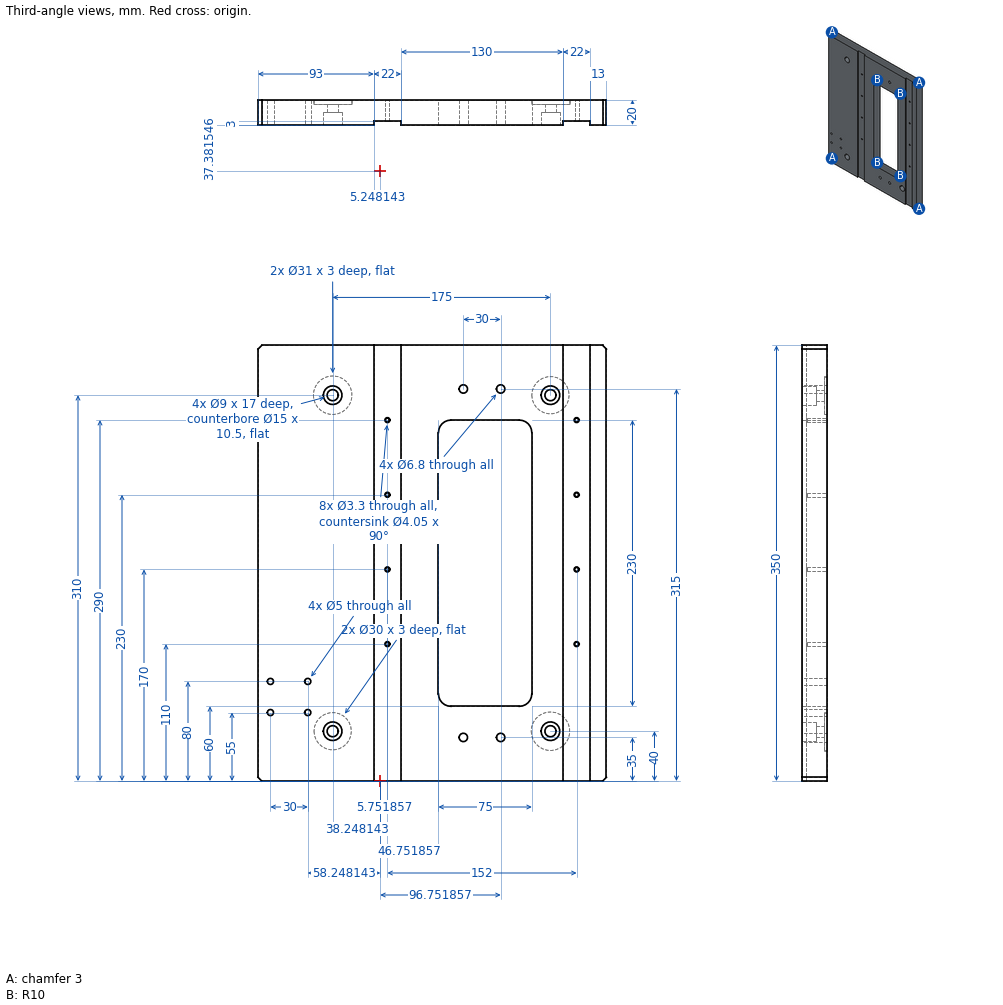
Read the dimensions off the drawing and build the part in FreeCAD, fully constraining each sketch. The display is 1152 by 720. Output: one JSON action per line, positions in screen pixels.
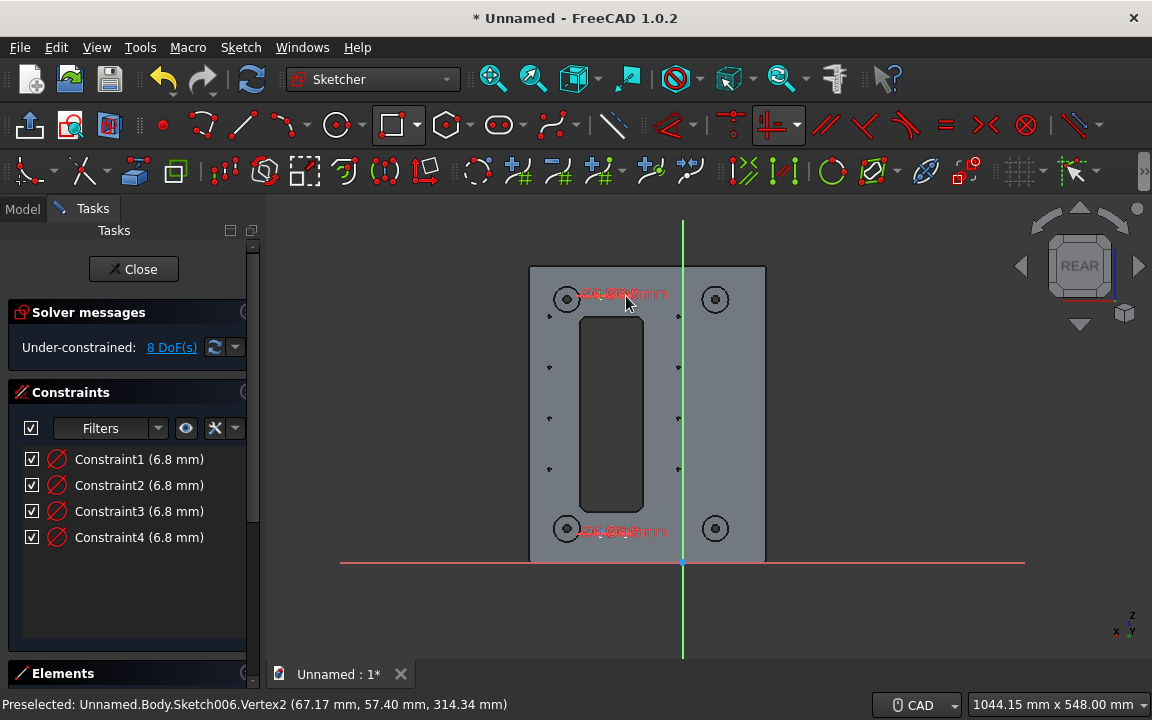
{"action": "left_click", "coordinate": [800, 126]}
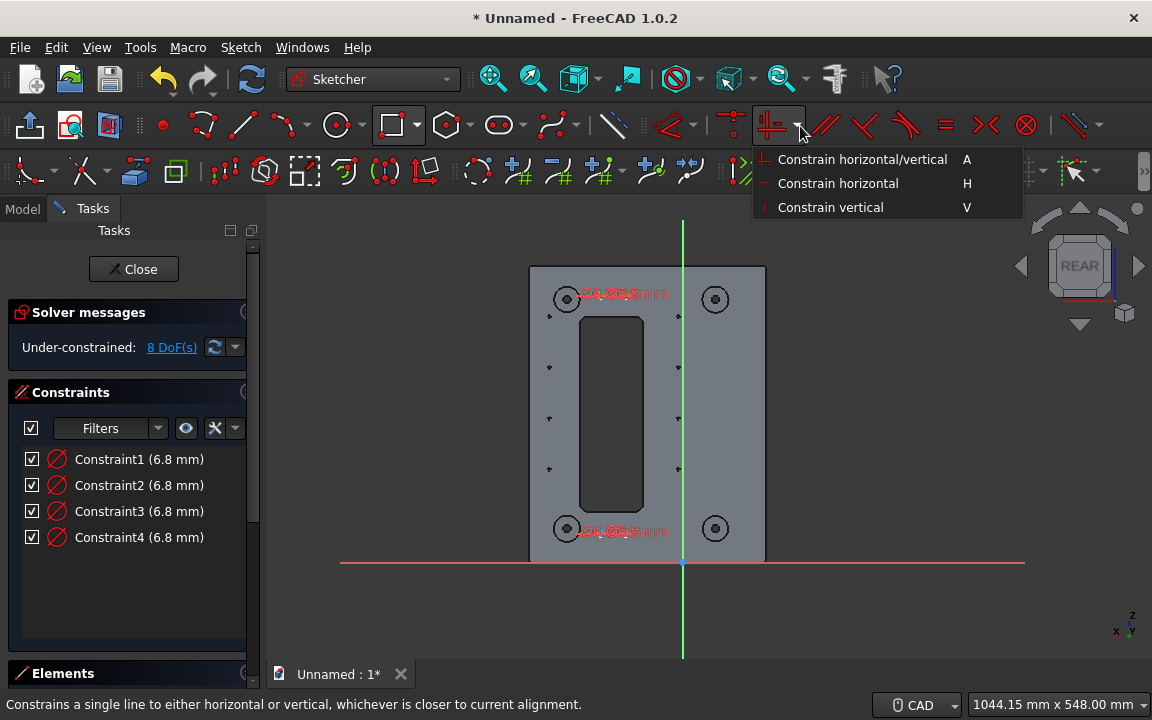
{"action": "left_click", "coordinate": [888, 183]}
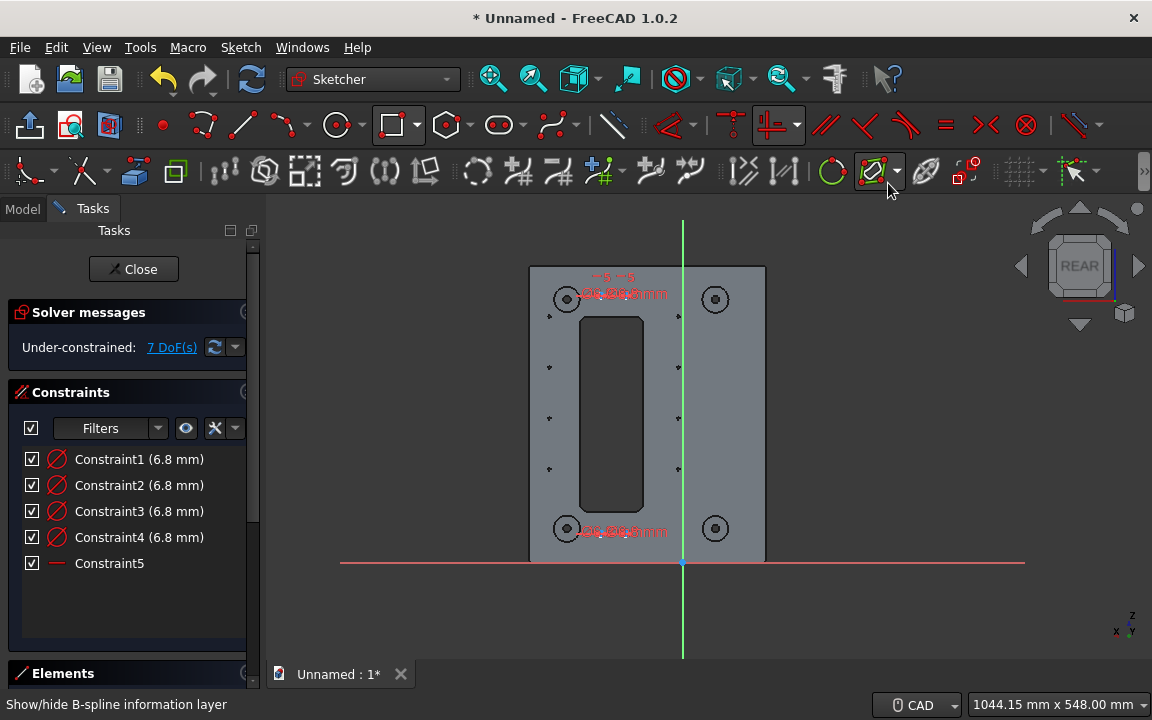
{"action": "left_click", "coordinate": [601, 296]}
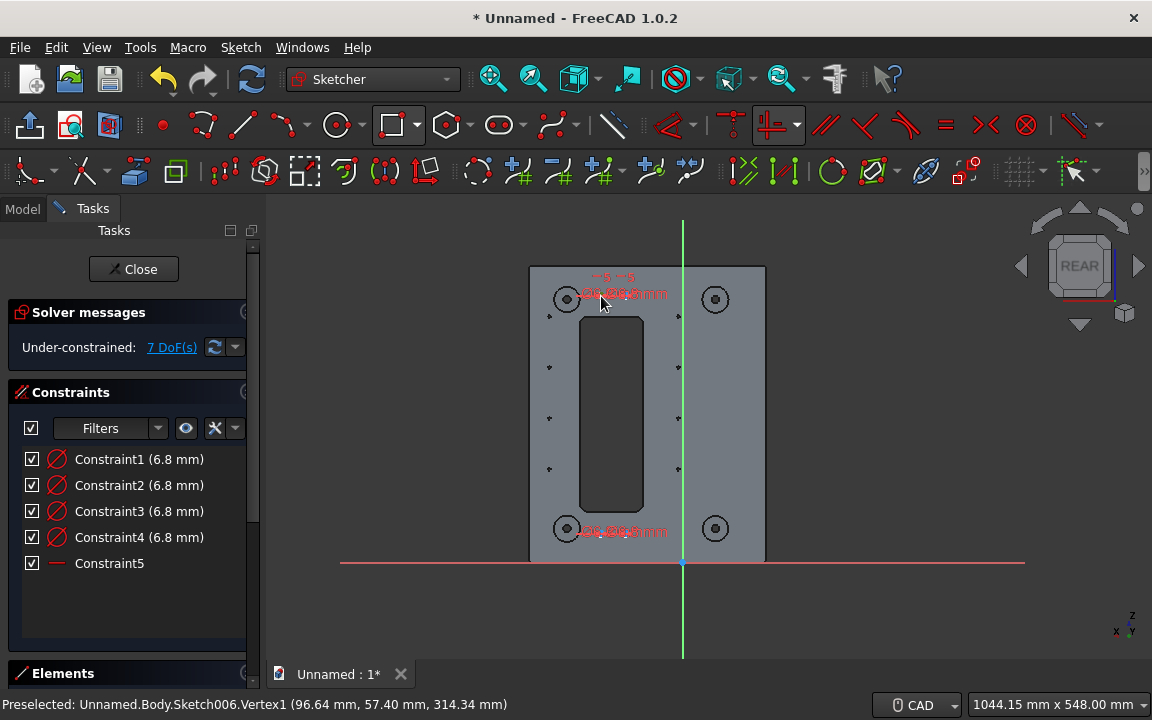
{"action": "left_click", "coordinate": [601, 534]}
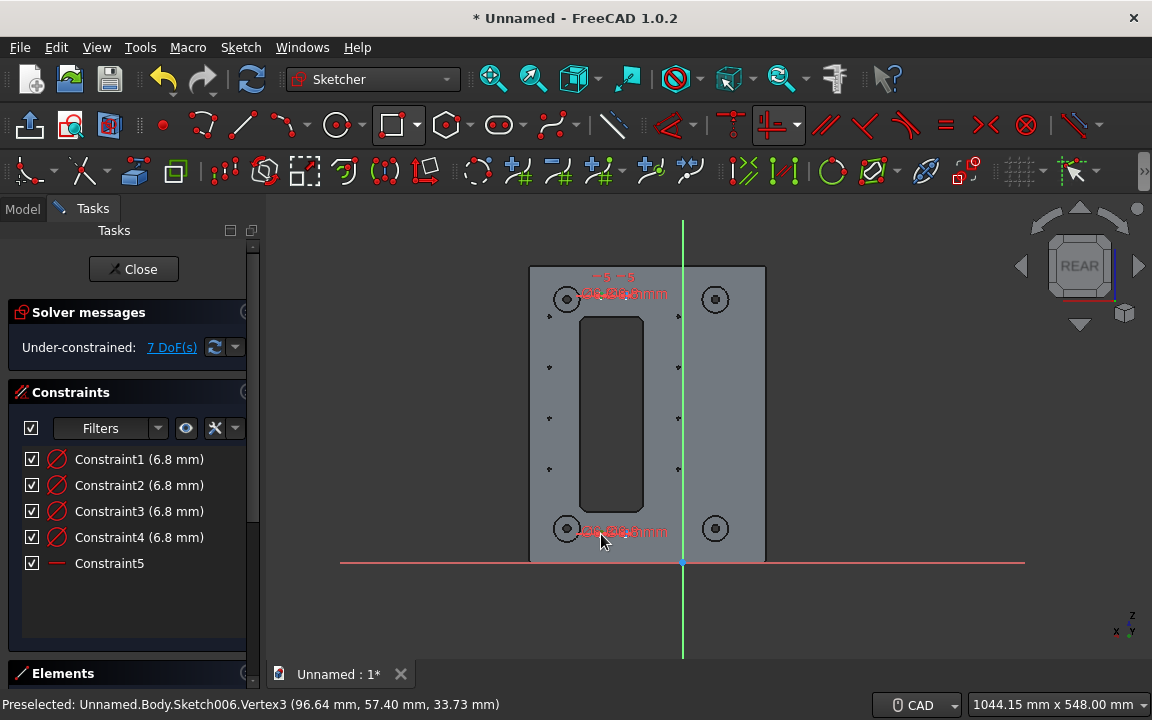
{"action": "key", "text": "v"}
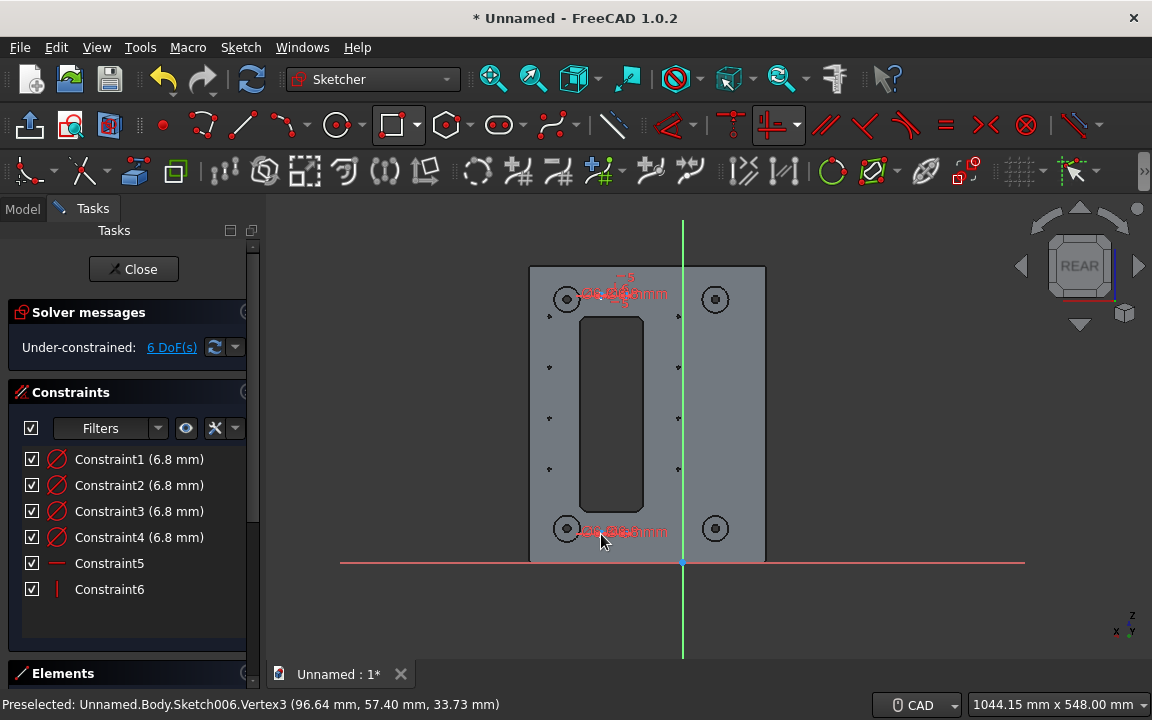
{"action": "left_click", "coordinate": [626, 296]}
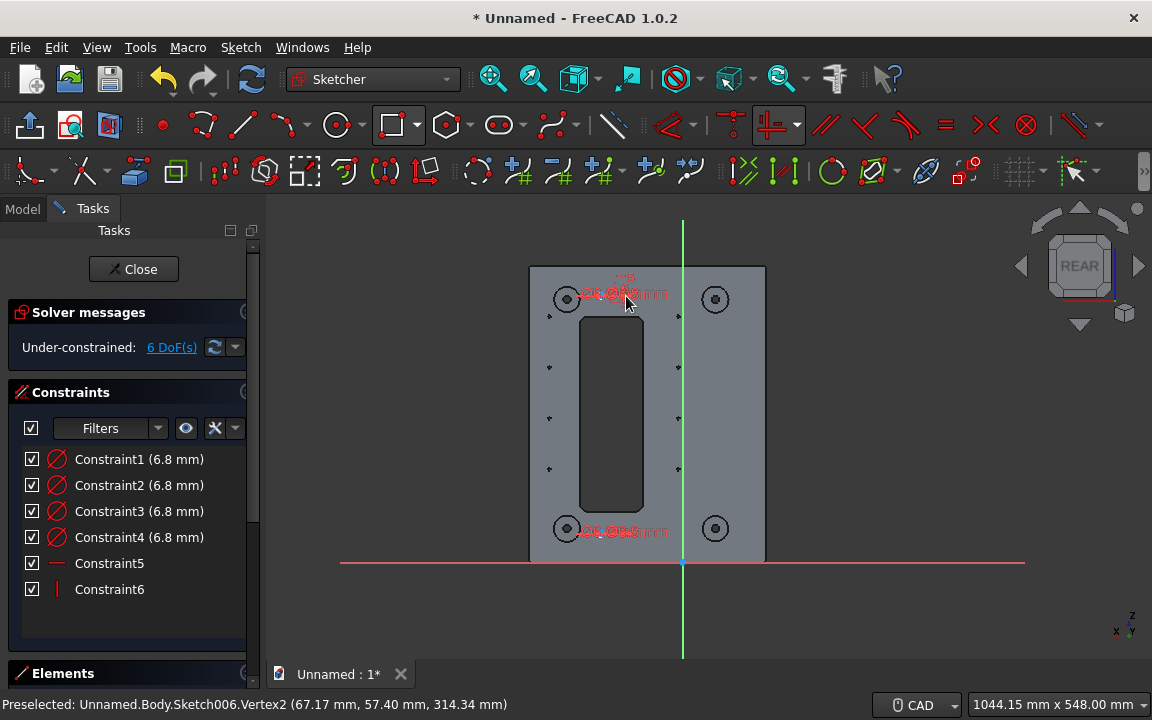
{"action": "scroll", "coordinate": [626, 534], "scroll_direction": "up", "scroll_amount": 4}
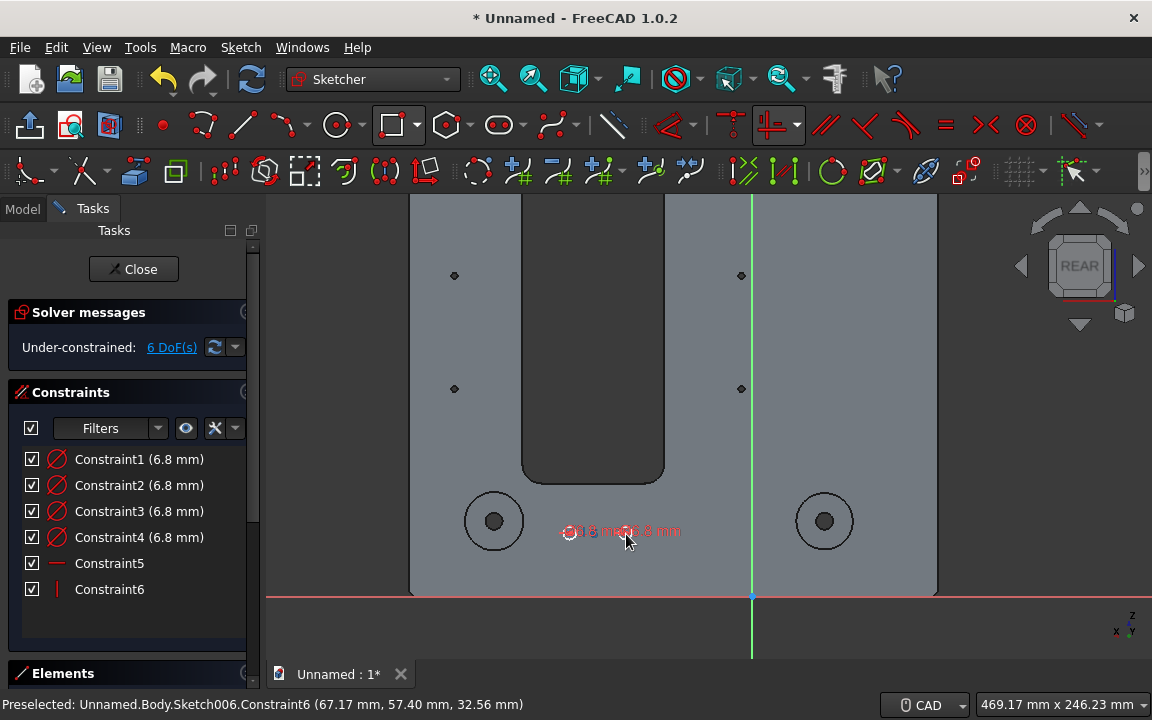
{"action": "left_click", "coordinate": [626, 533]}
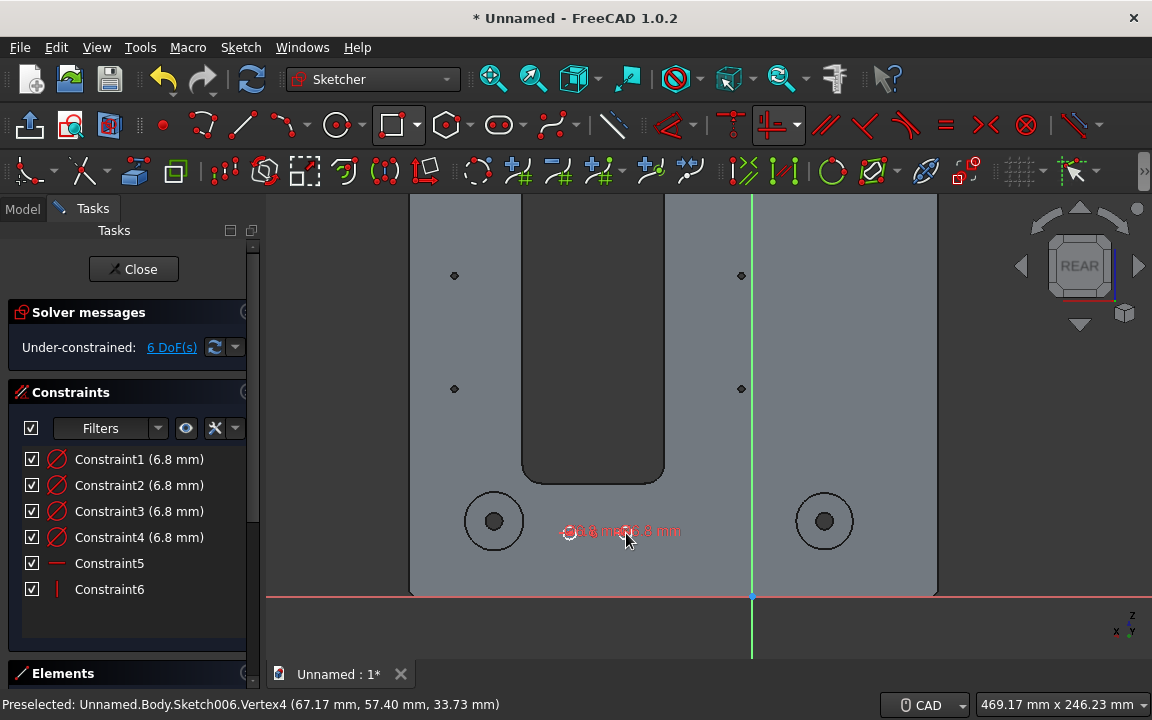
{"action": "left_click", "coordinate": [800, 126]}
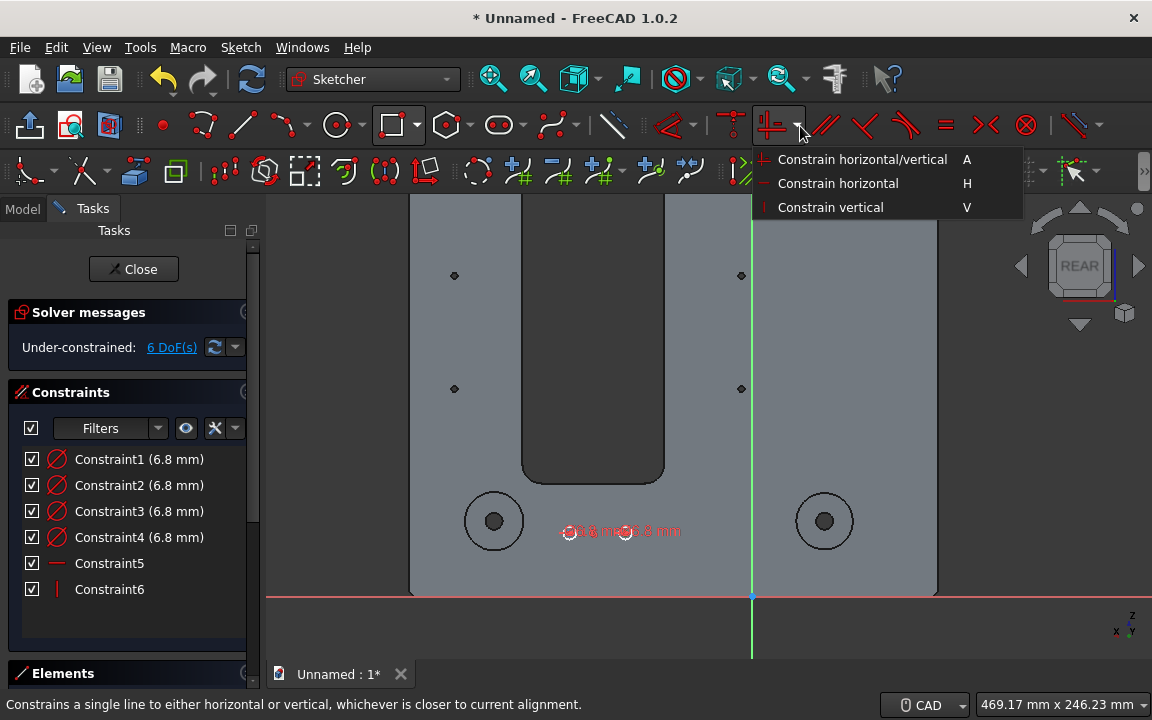
{"action": "left_click", "coordinate": [888, 207]}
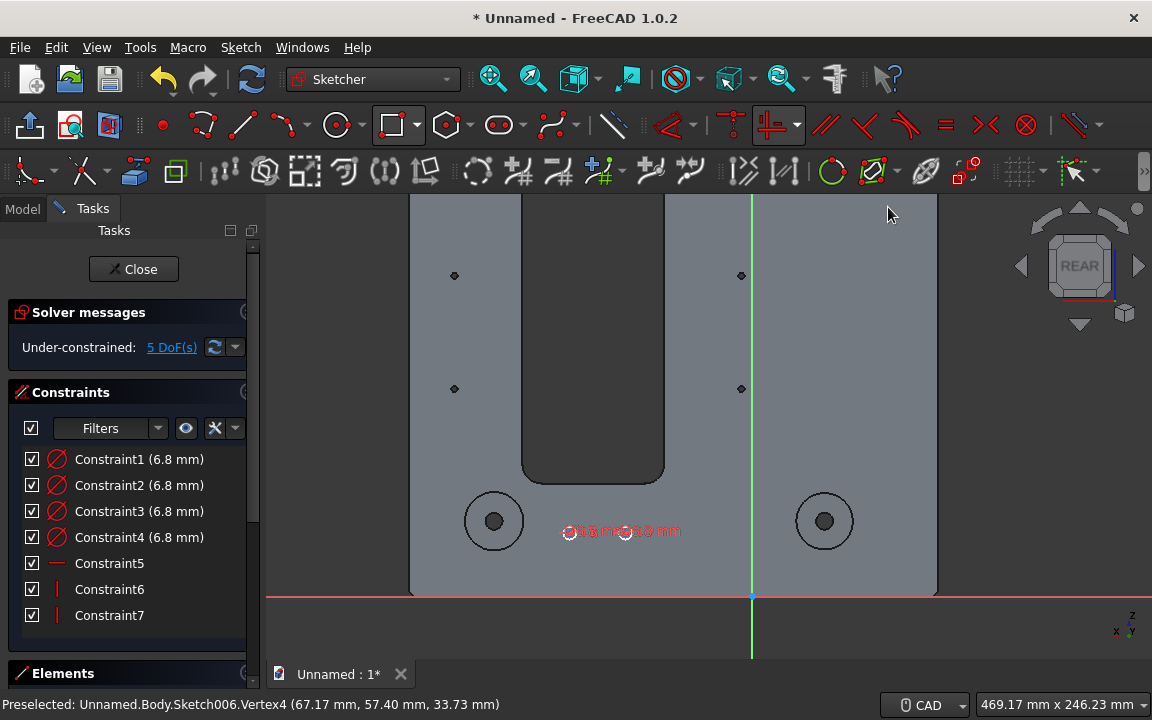
{"action": "left_click", "coordinate": [570, 533]}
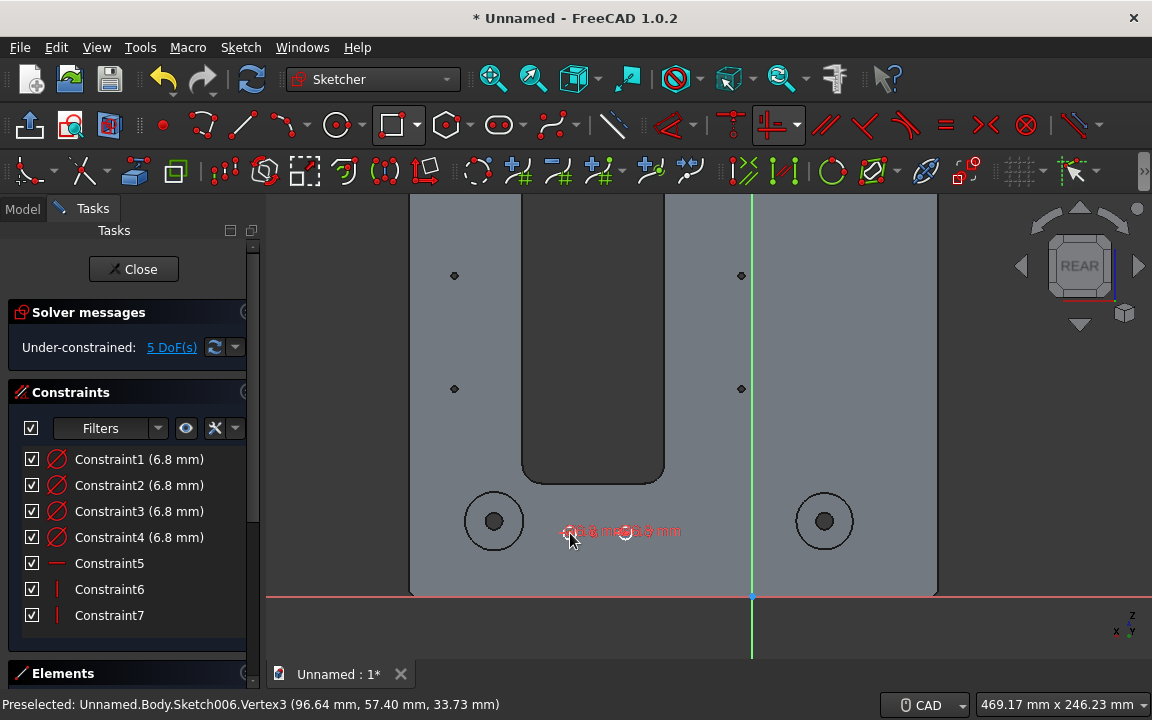
{"action": "left_click", "coordinate": [626, 533]}